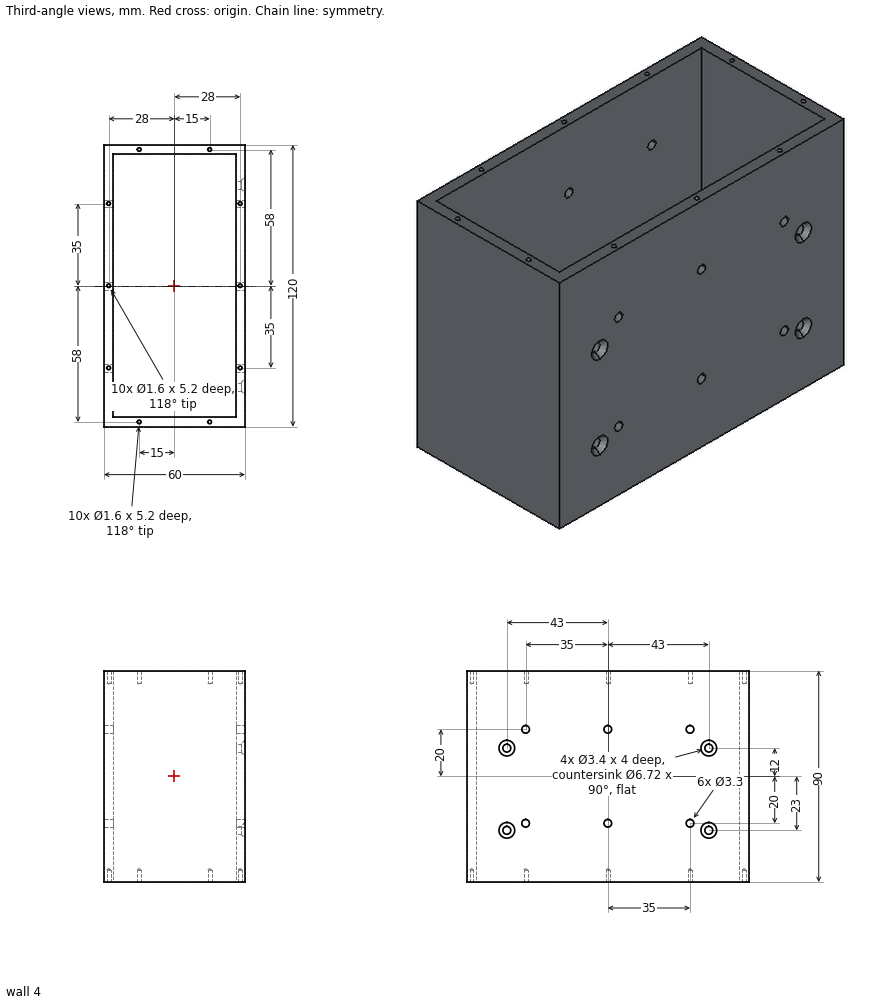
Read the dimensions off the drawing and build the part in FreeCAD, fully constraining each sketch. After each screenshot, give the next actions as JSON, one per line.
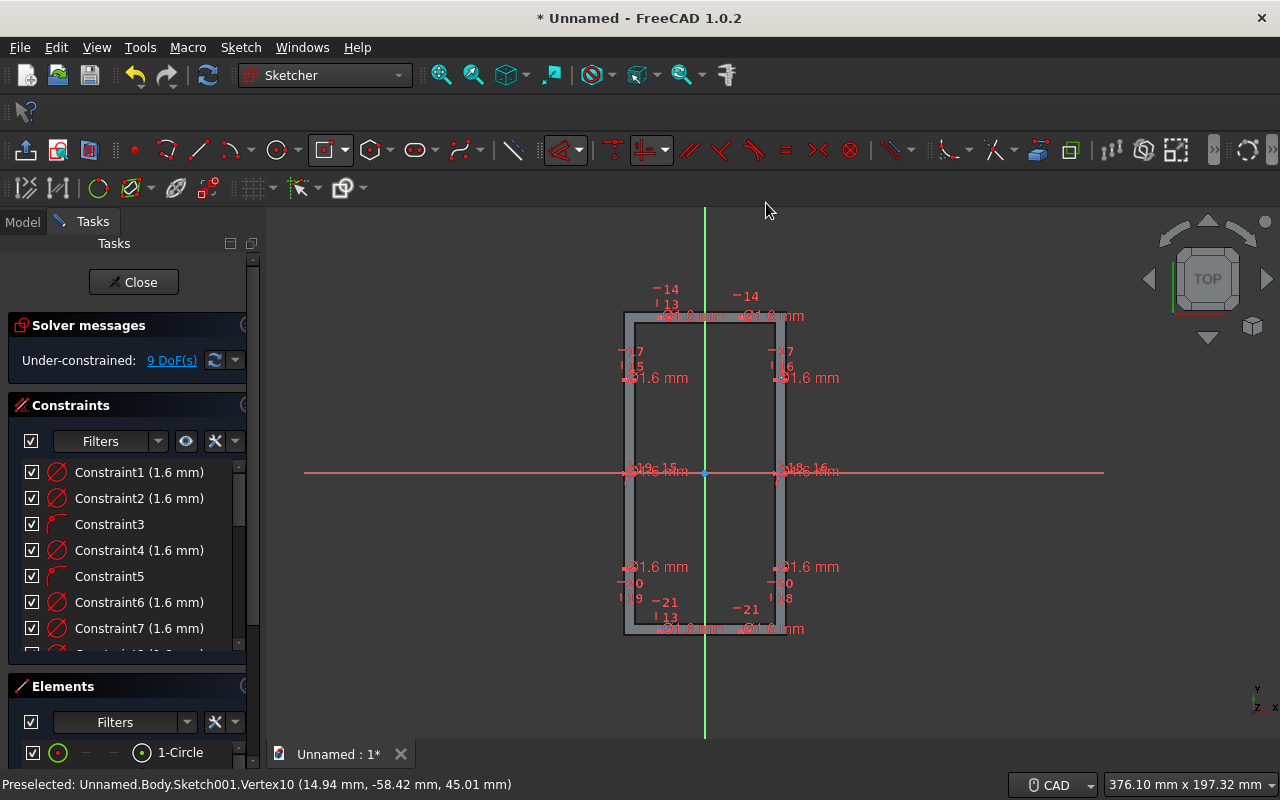
{"action": "left_click", "coordinate": [745, 318]}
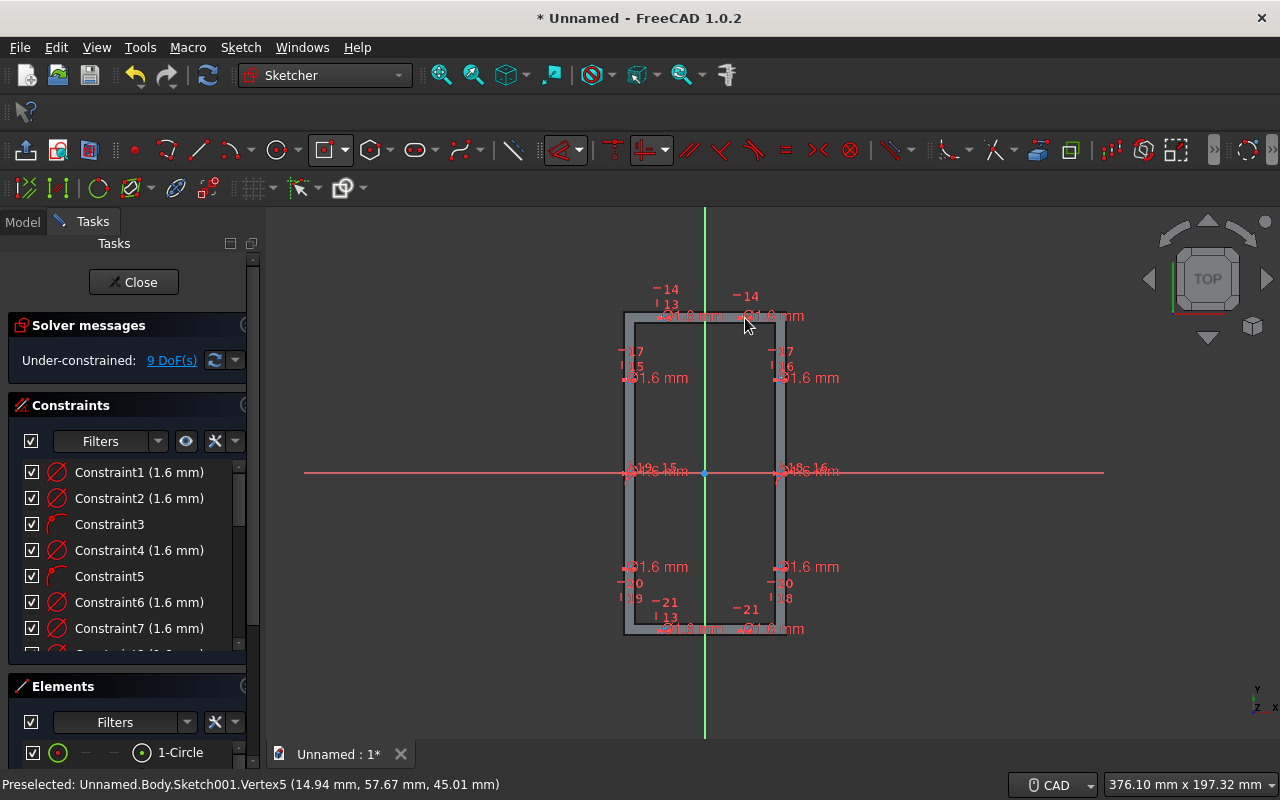
{"action": "left_click", "coordinate": [745, 631]}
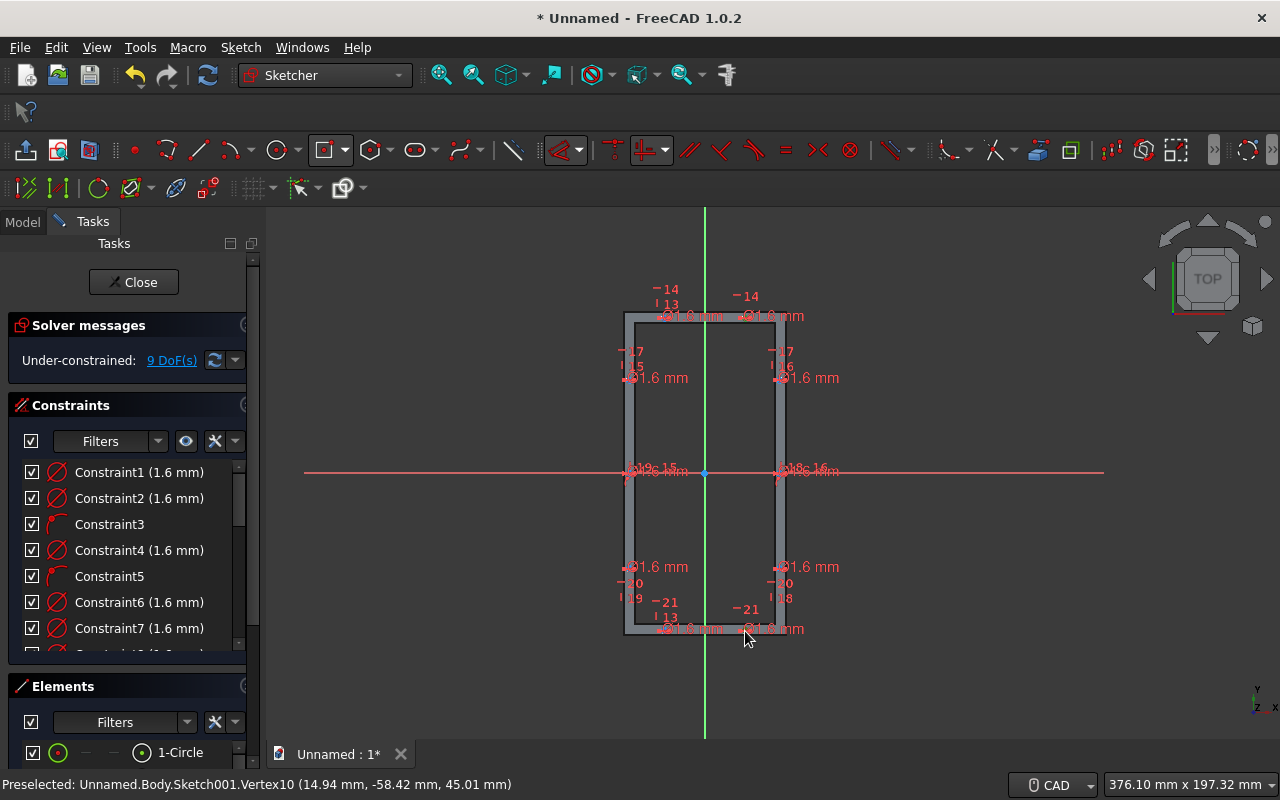
{"action": "left_click", "coordinate": [353, 473]}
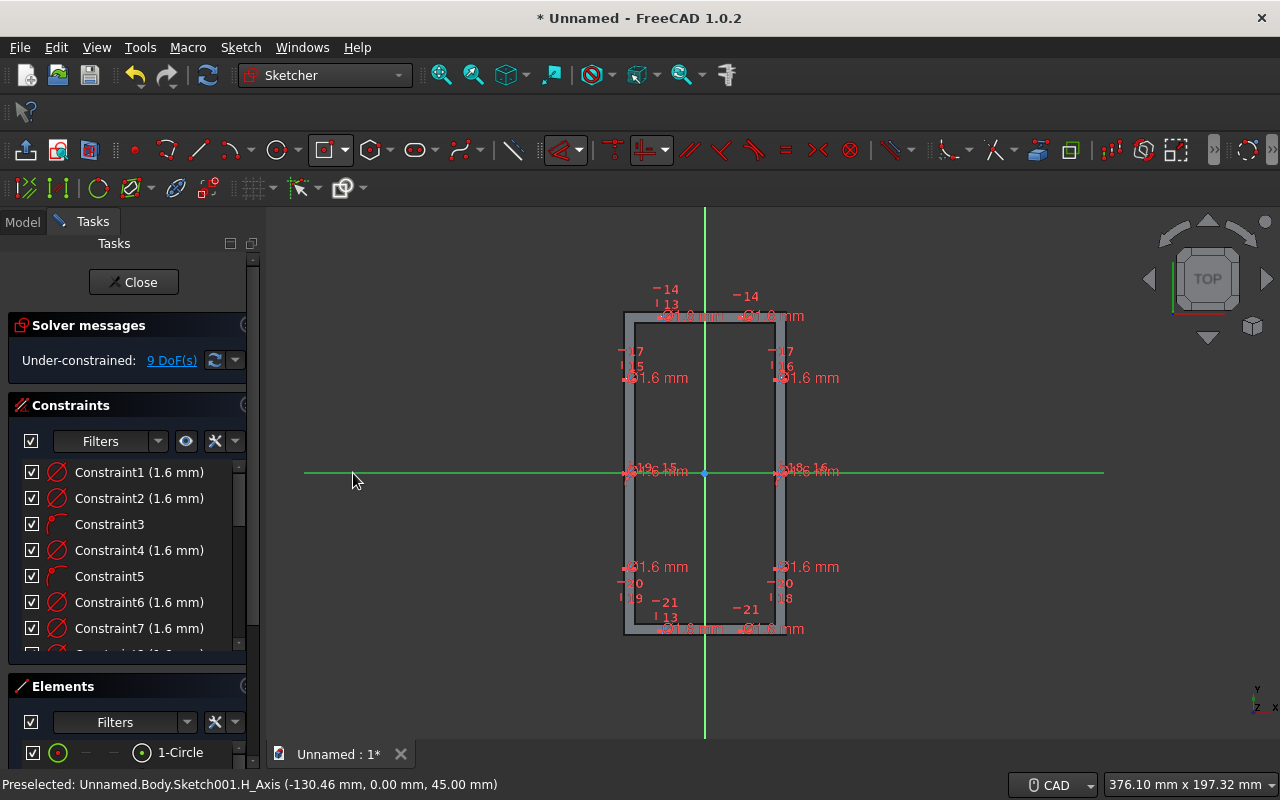
{"action": "left_click", "coordinate": [818, 150]}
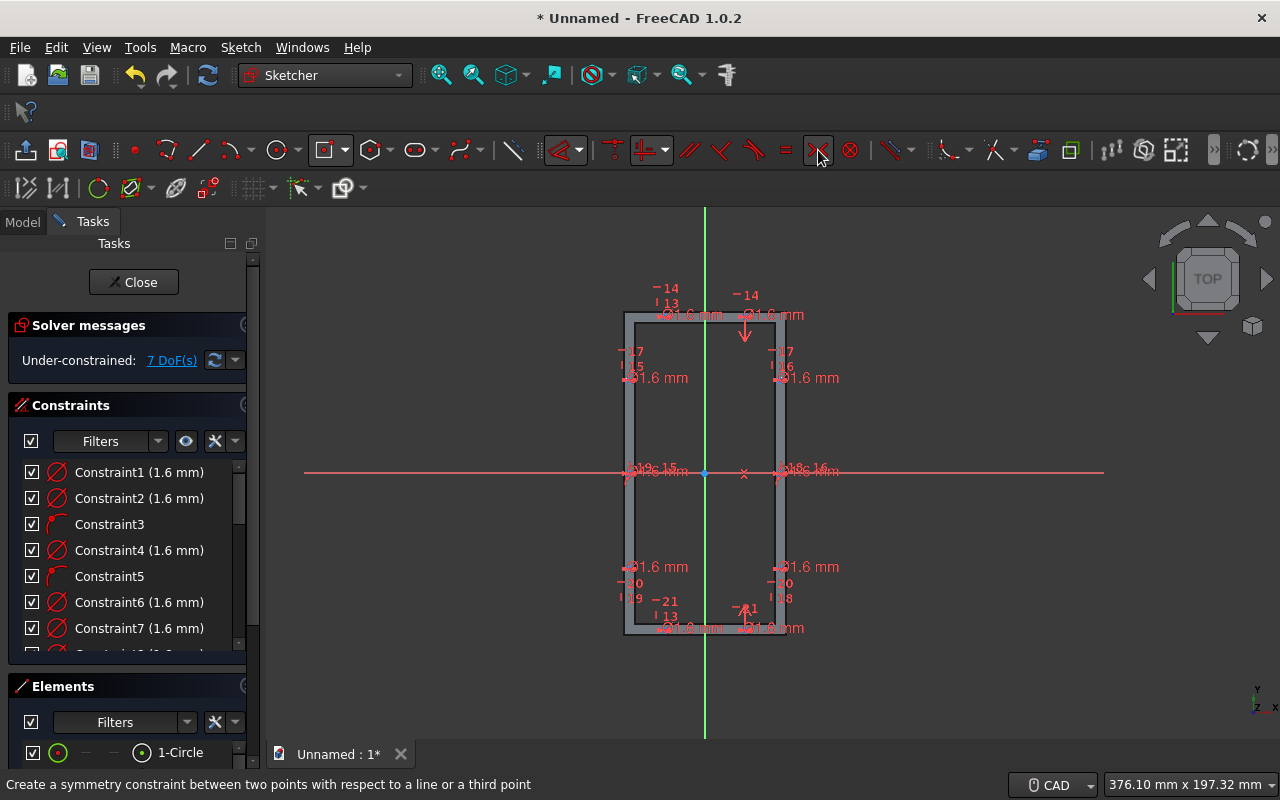
{"action": "left_click", "coordinate": [560, 150]}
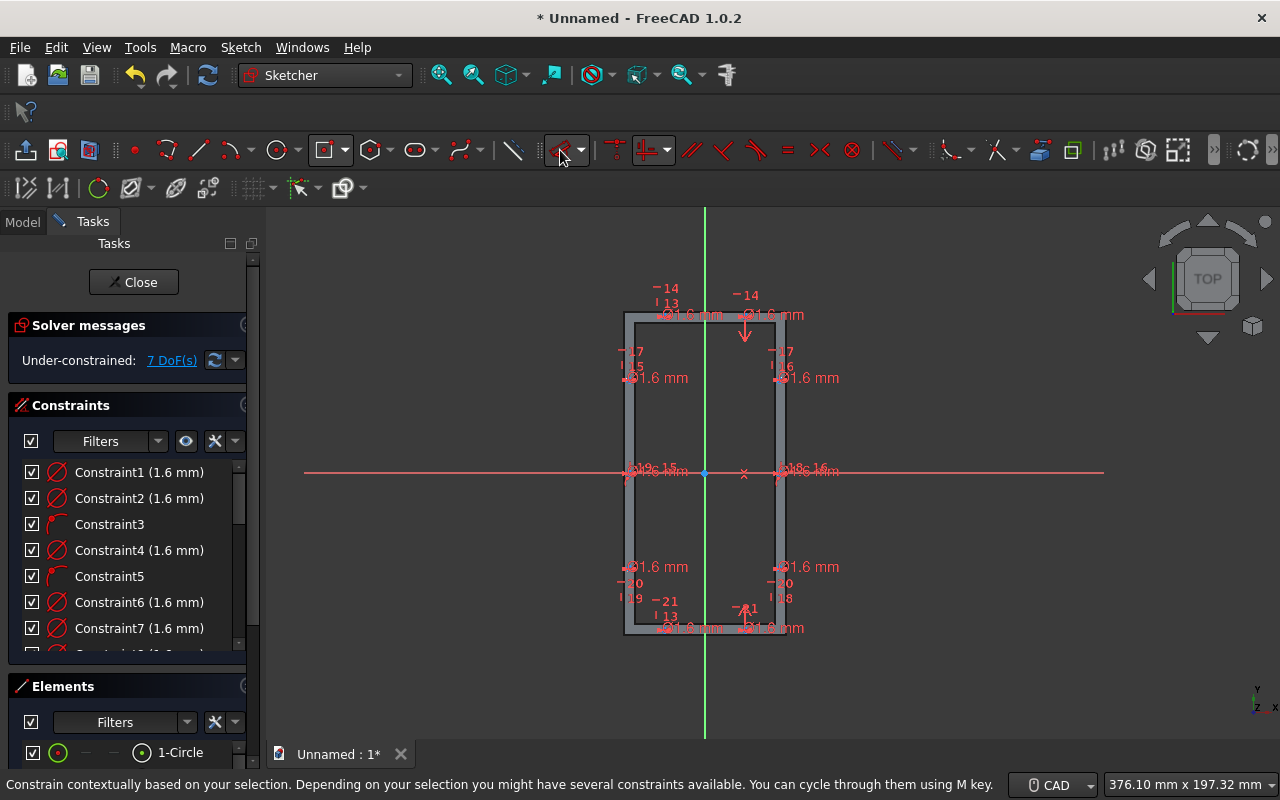
{"action": "left_click", "coordinate": [664, 630]}
{"action": "left_click", "coordinate": [684, 664]}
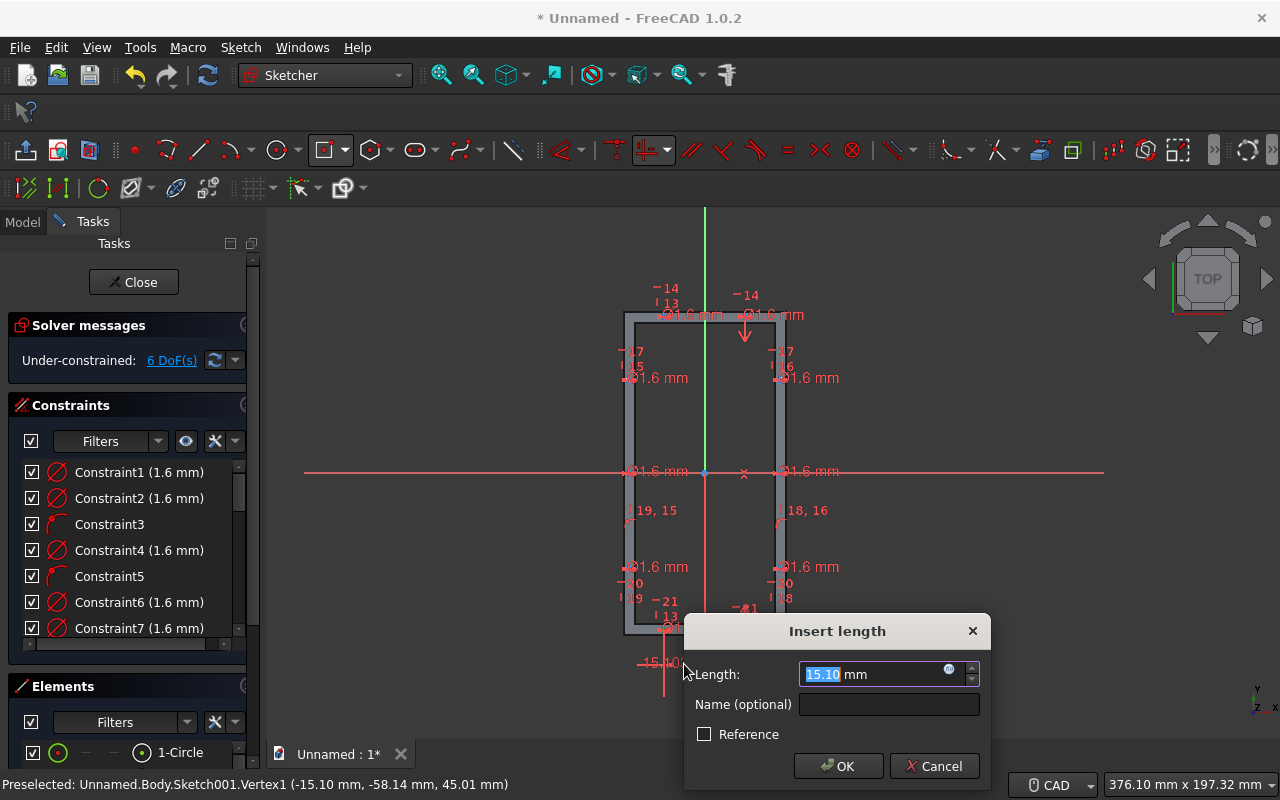
{"action": "type", "text": "15"}
{"action": "key", "text": "Return"}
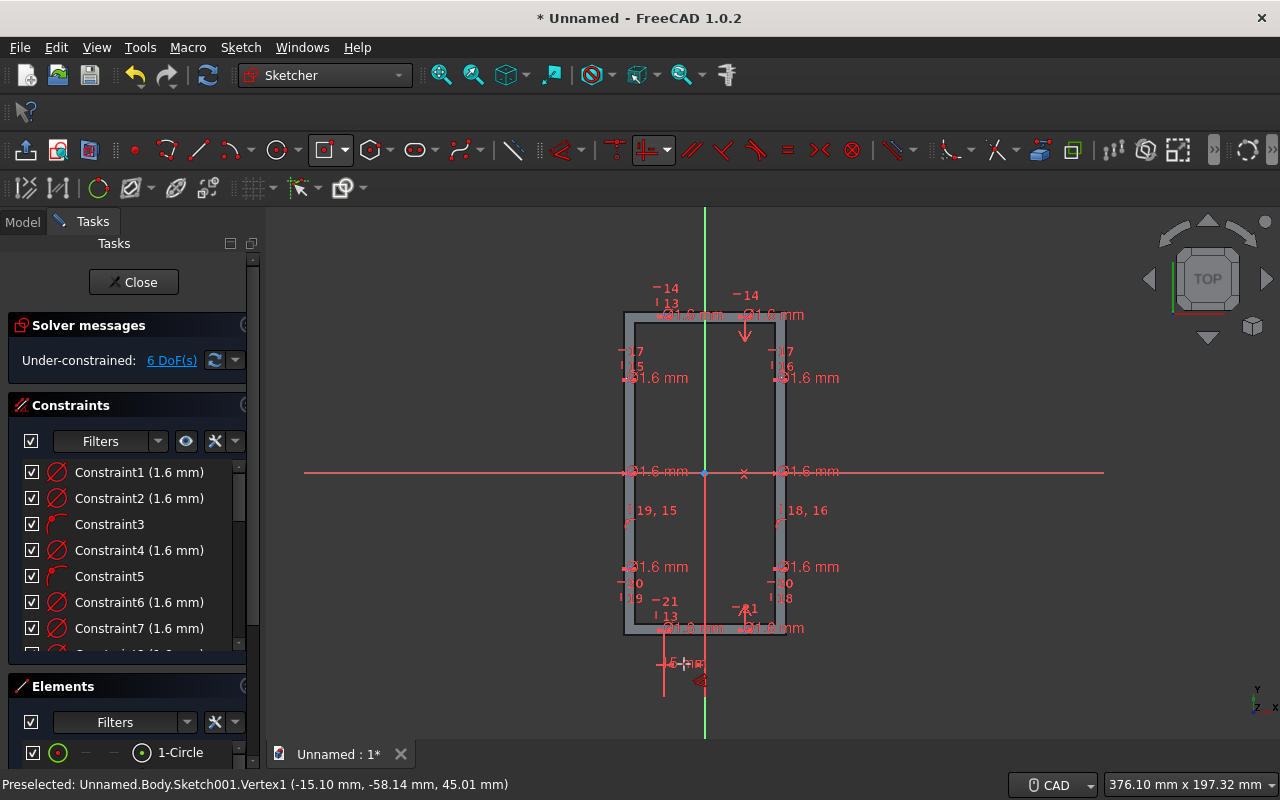
{"action": "left_click", "coordinate": [664, 630]}
{"action": "left_click", "coordinate": [630, 552]}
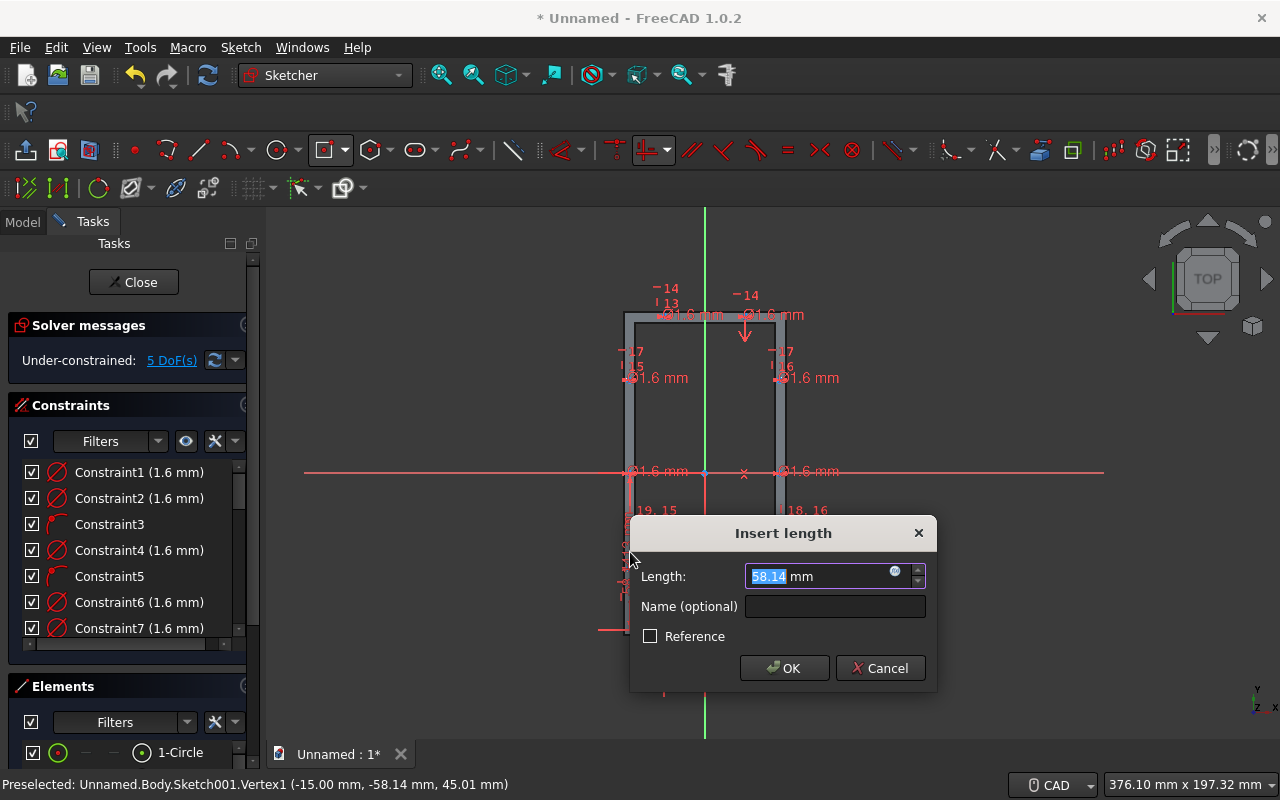
{"action": "type", "text": "58"}
{"action": "key", "text": "Return"}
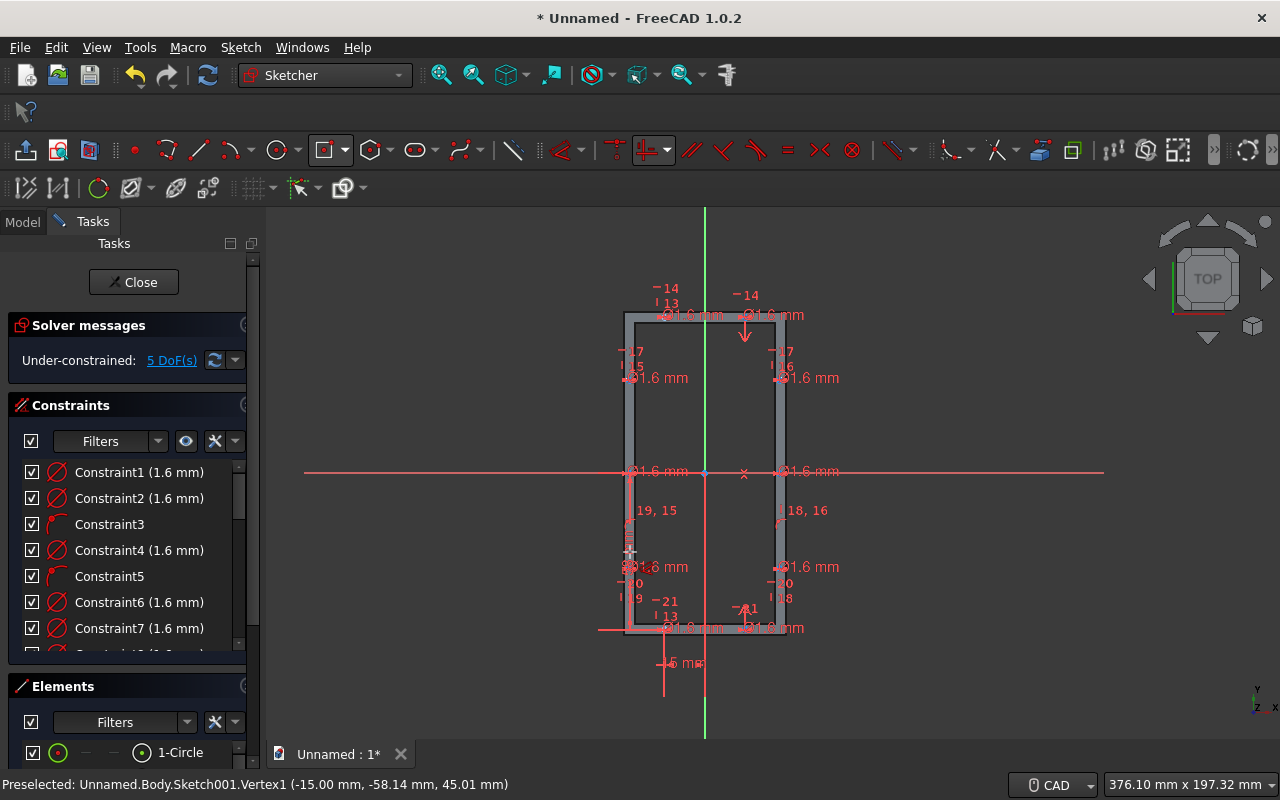
{"action": "left_click", "coordinate": [629, 473]}
{"action": "left_click", "coordinate": [667, 507]}